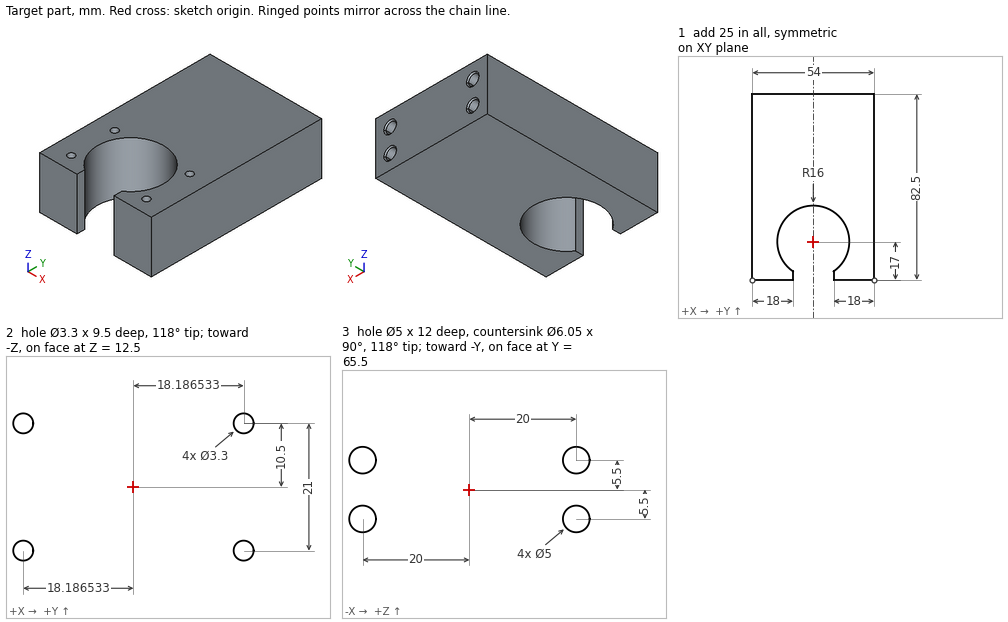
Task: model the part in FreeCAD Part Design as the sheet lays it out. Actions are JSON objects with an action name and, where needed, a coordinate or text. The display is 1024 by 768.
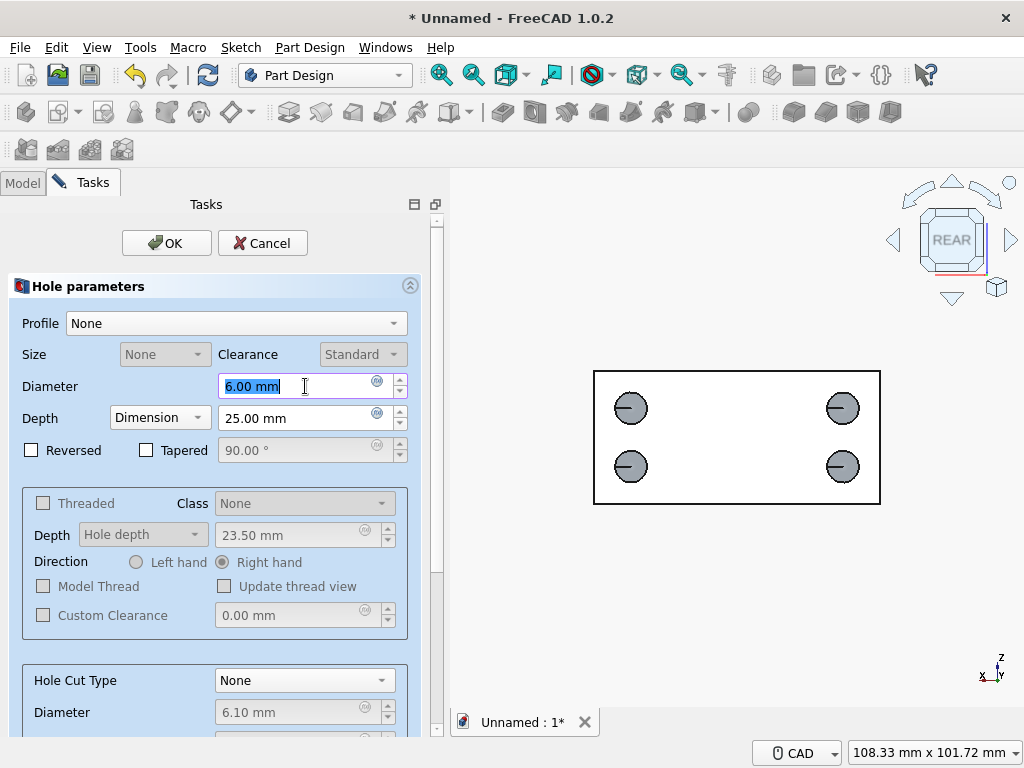
{"action": "type", "text": "5"}
{"action": "key", "text": "Tab"}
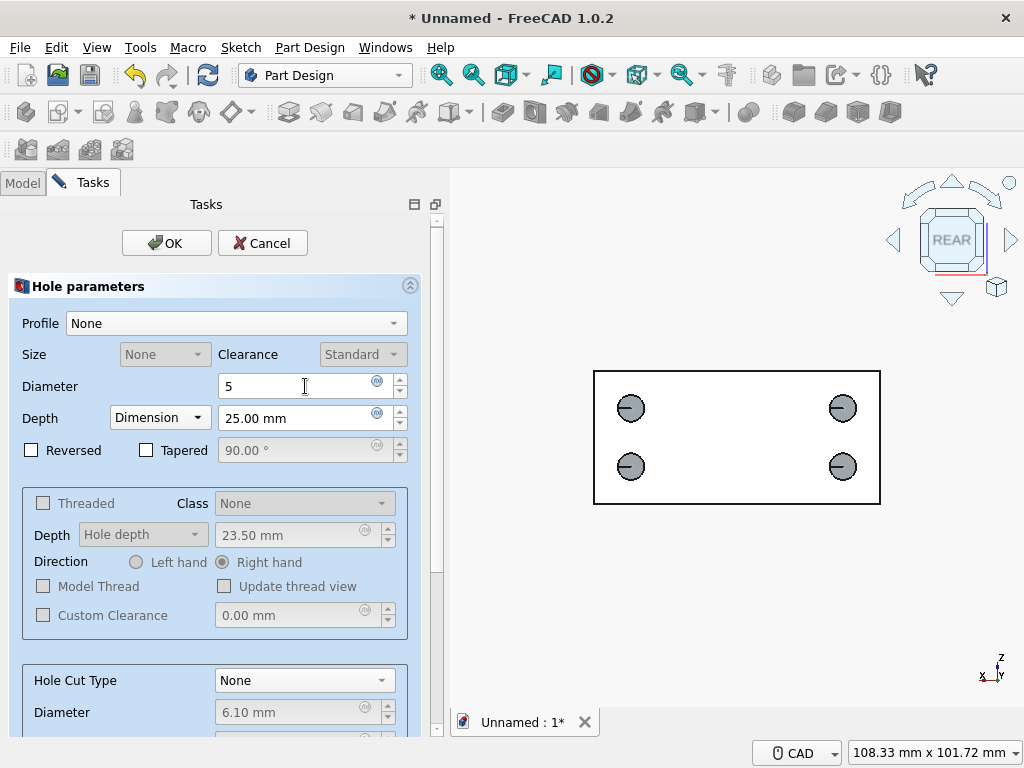
{"action": "triple_click", "coordinate": [305, 418]}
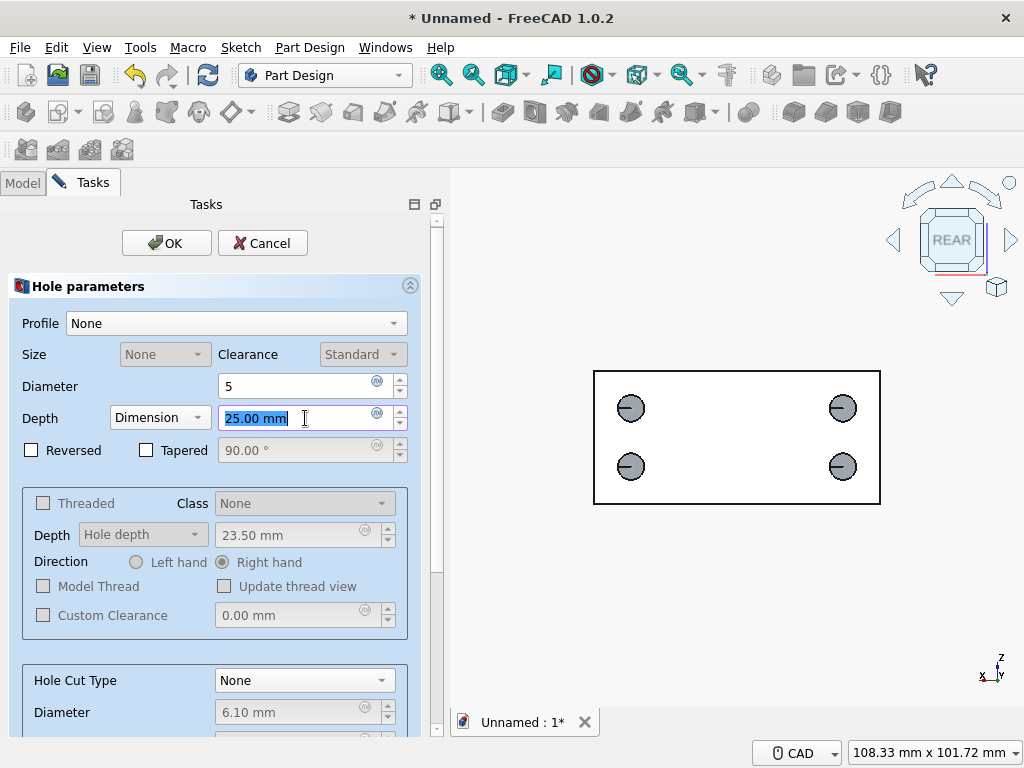
{"action": "type", "text": "12"}
{"action": "key", "text": "Tab"}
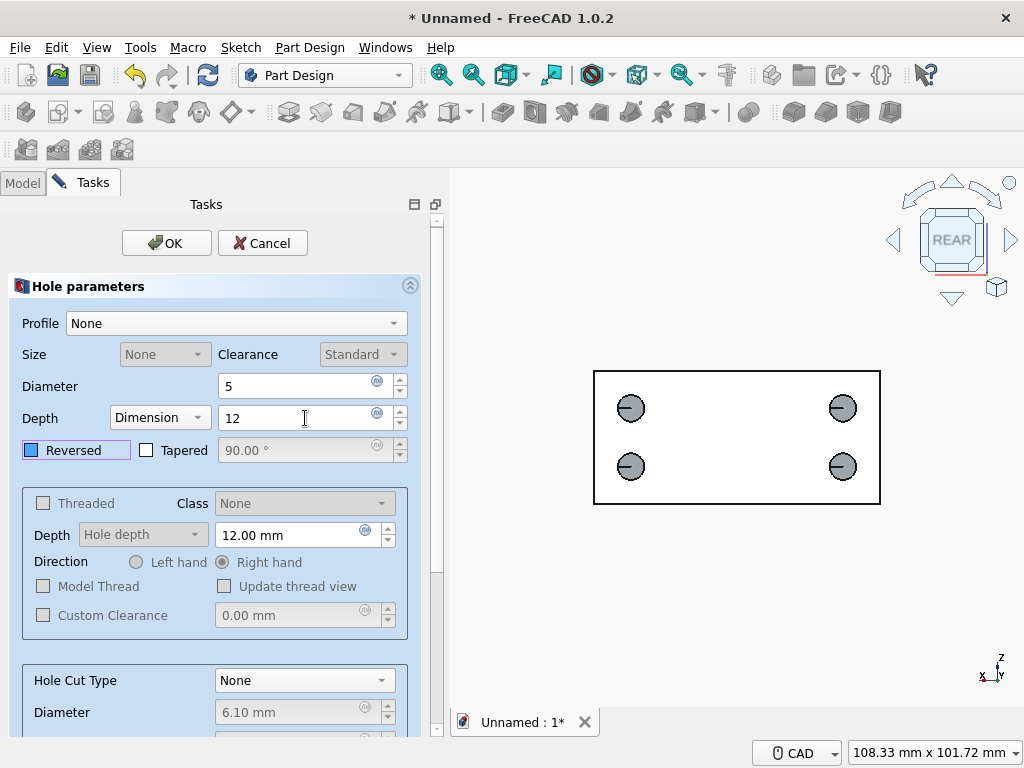
{"action": "left_click", "coordinate": [306, 680]}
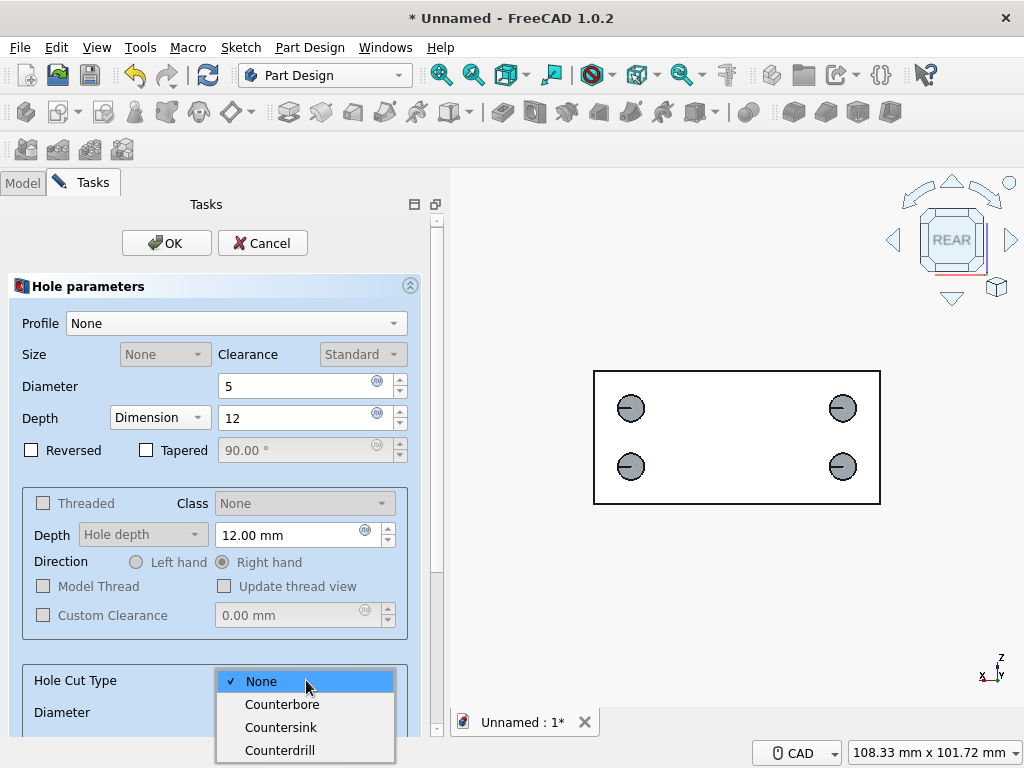
{"action": "left_click", "coordinate": [304, 728]}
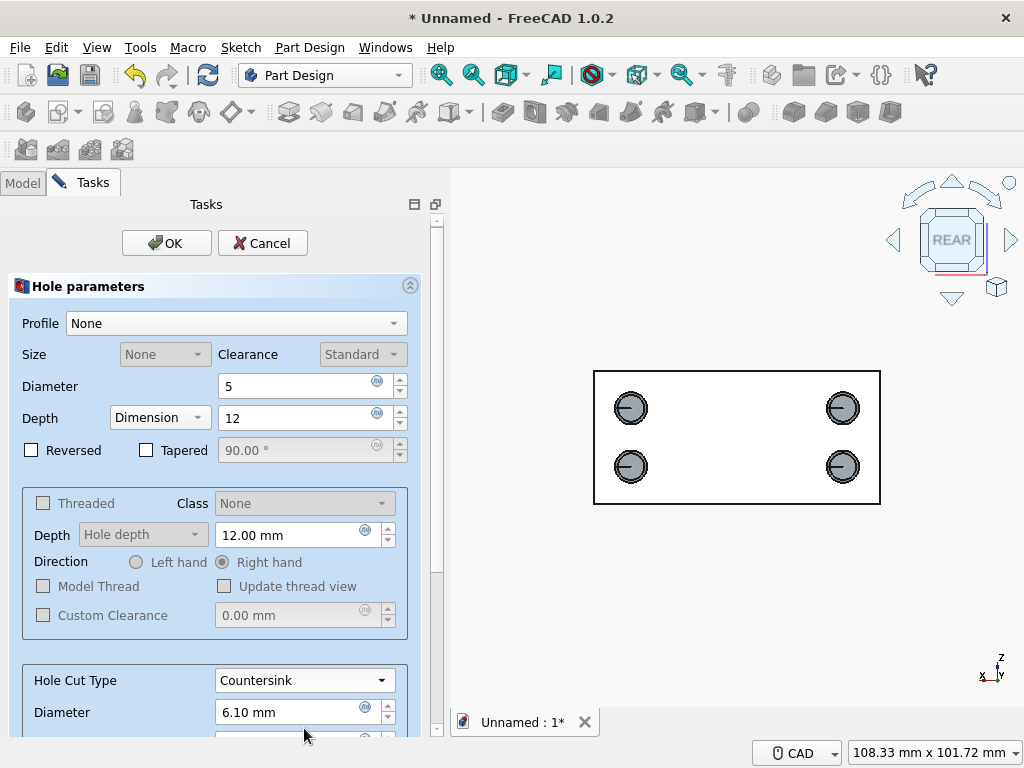
{"action": "triple_click", "coordinate": [298, 712]}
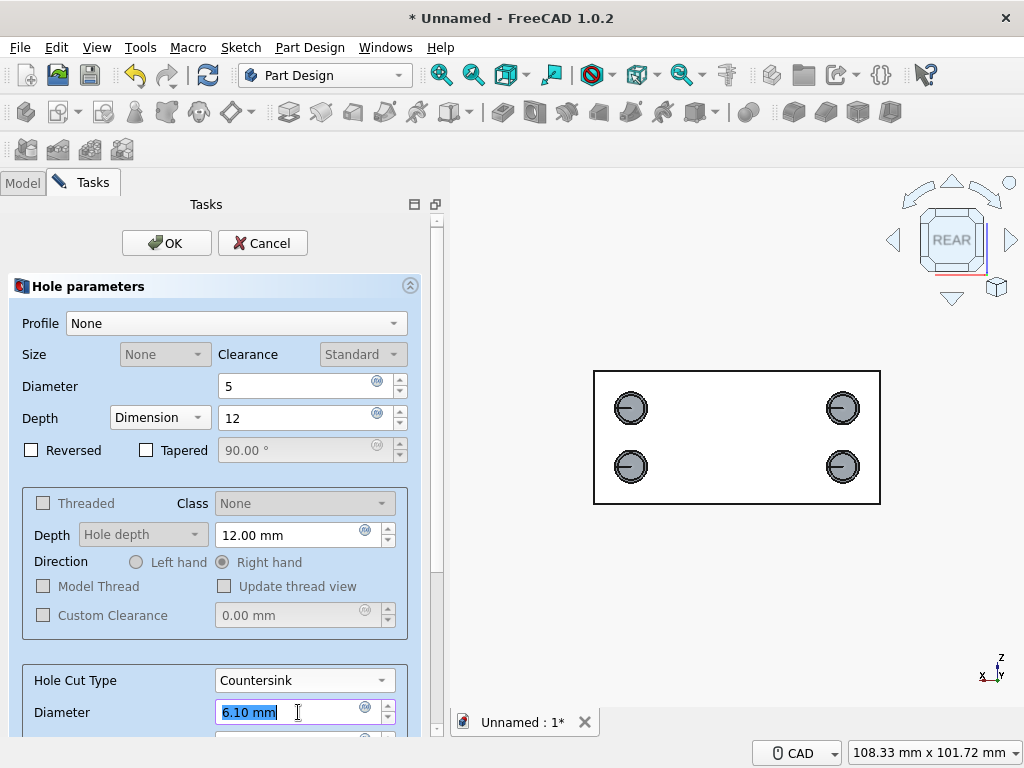
{"action": "type", "text": "6.05"}
{"action": "key", "text": "Tab"}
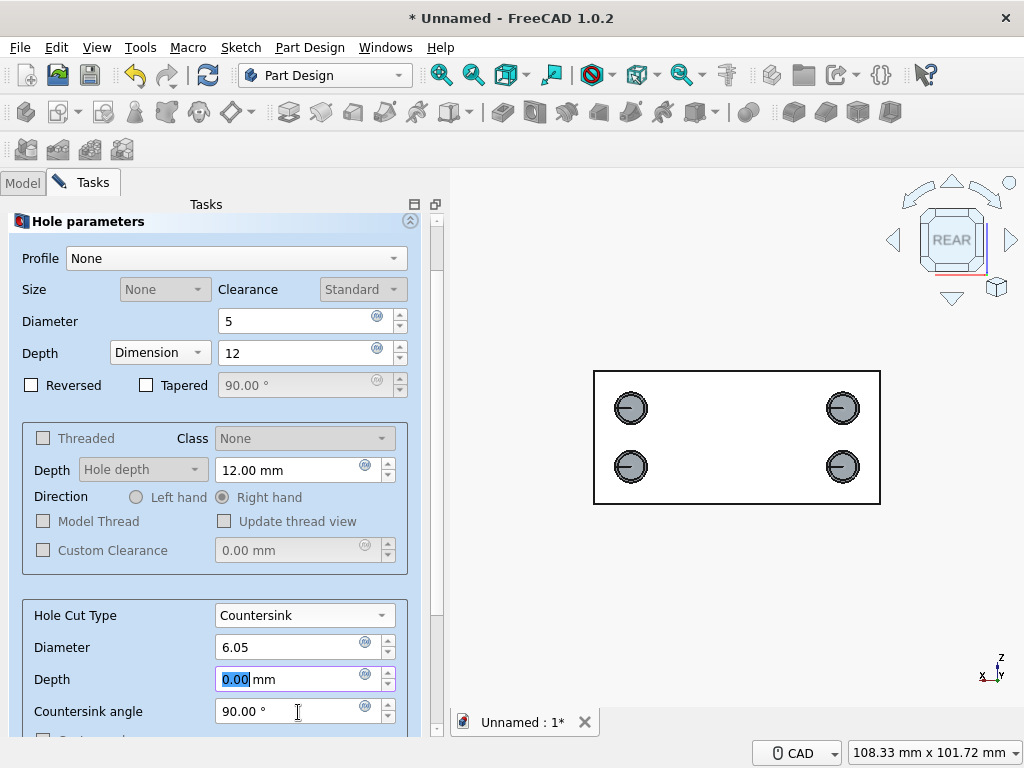
{"action": "scroll", "coordinate": [437, 475], "scroll_direction": "up", "scroll_amount": 2}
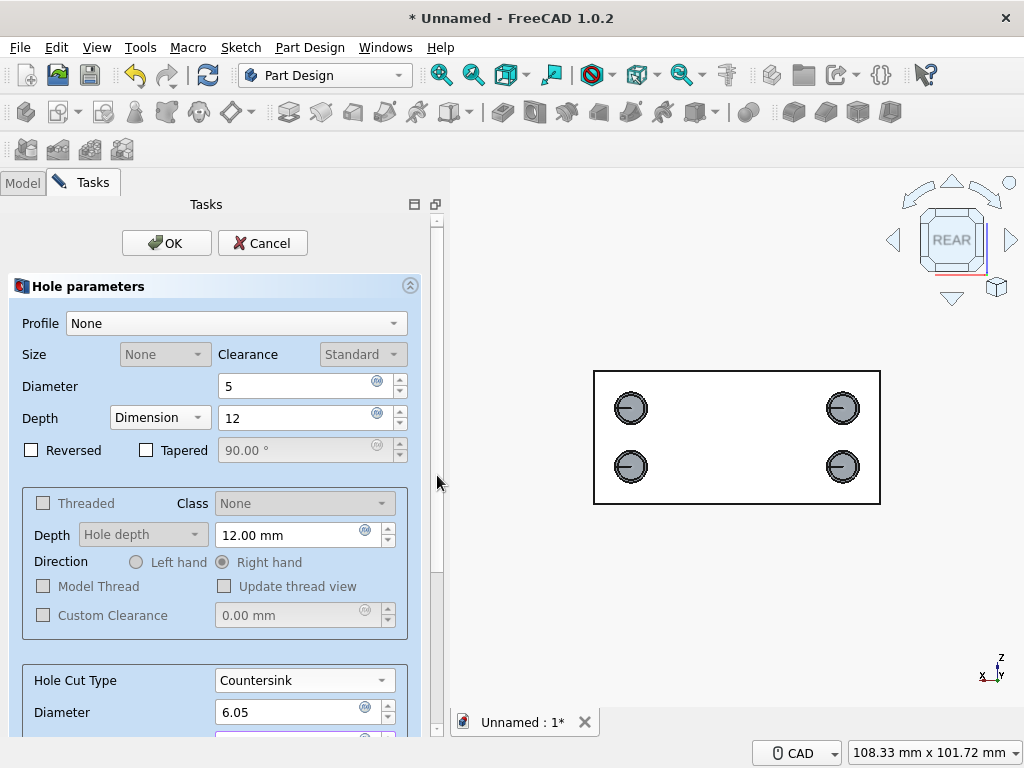
{"action": "left_click", "coordinate": [167, 243]}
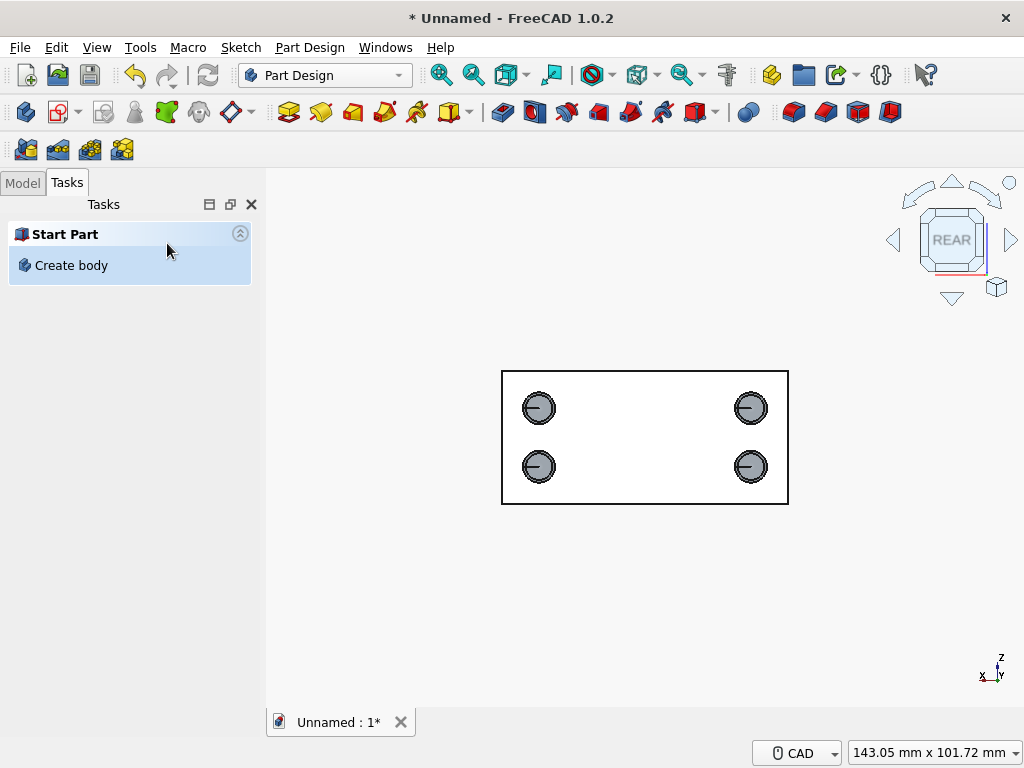
{"action": "key", "text": "0"}